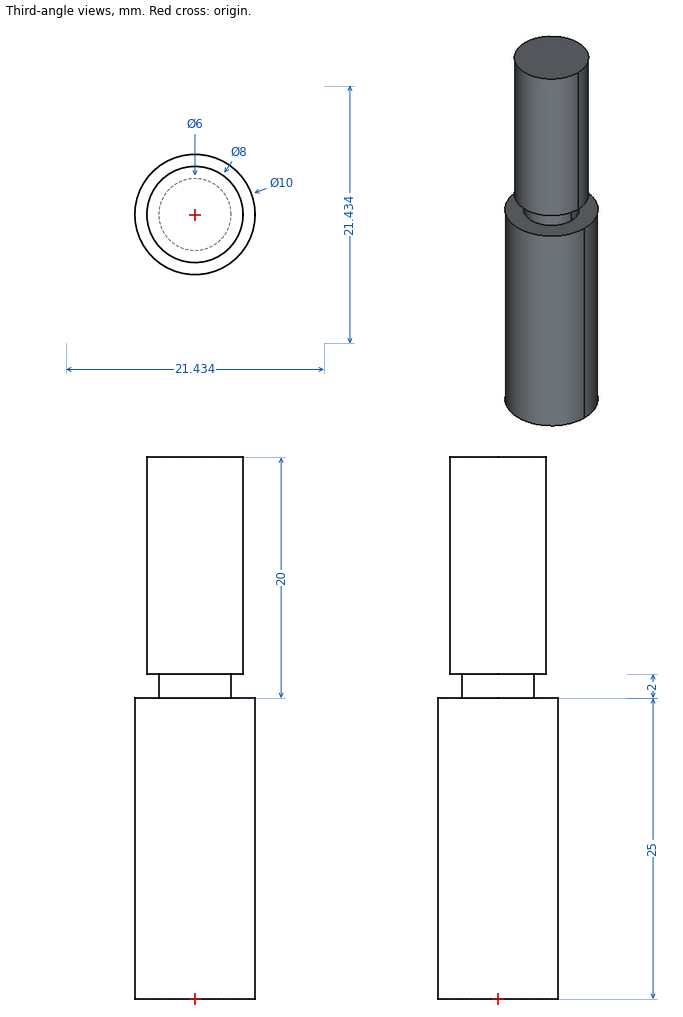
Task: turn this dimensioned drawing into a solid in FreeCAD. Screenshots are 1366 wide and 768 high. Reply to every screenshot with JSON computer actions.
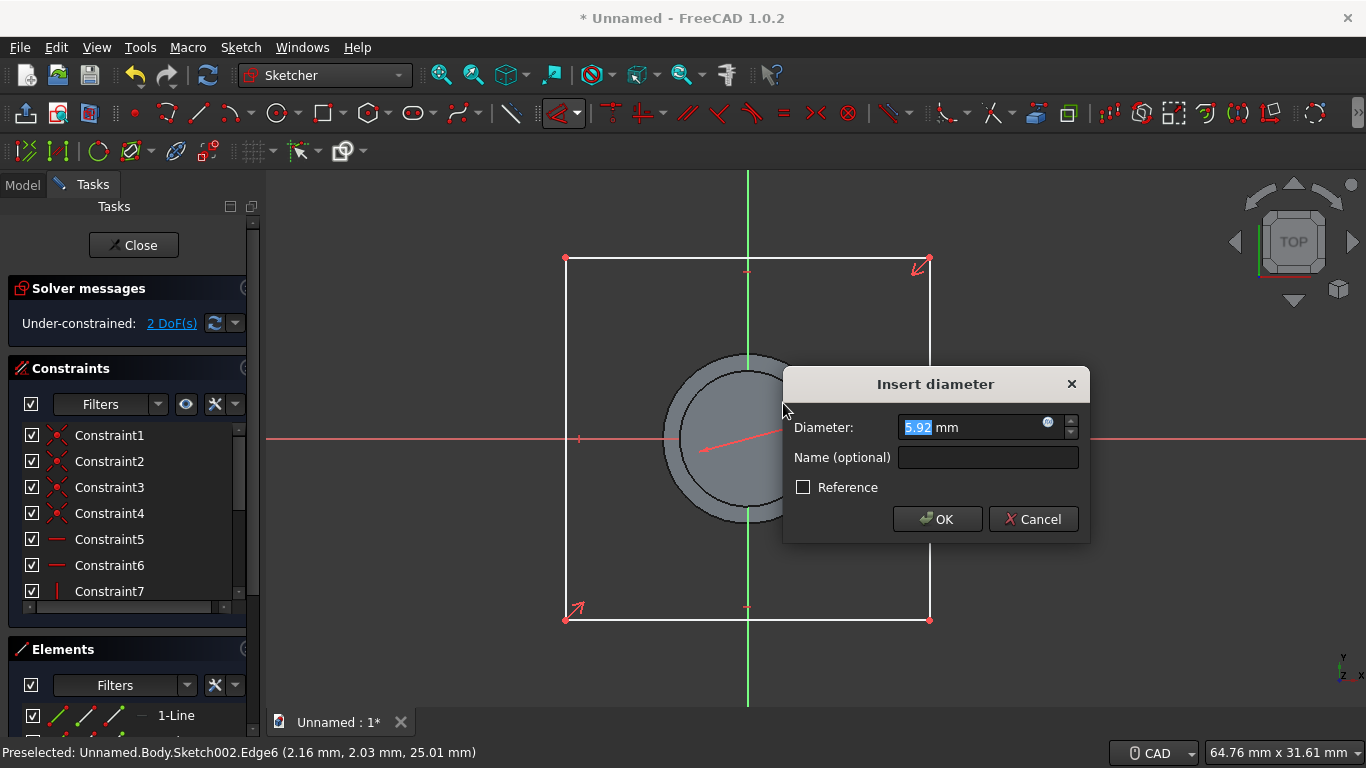
{"action": "type", "text": "6"}
{"action": "key", "text": "Return"}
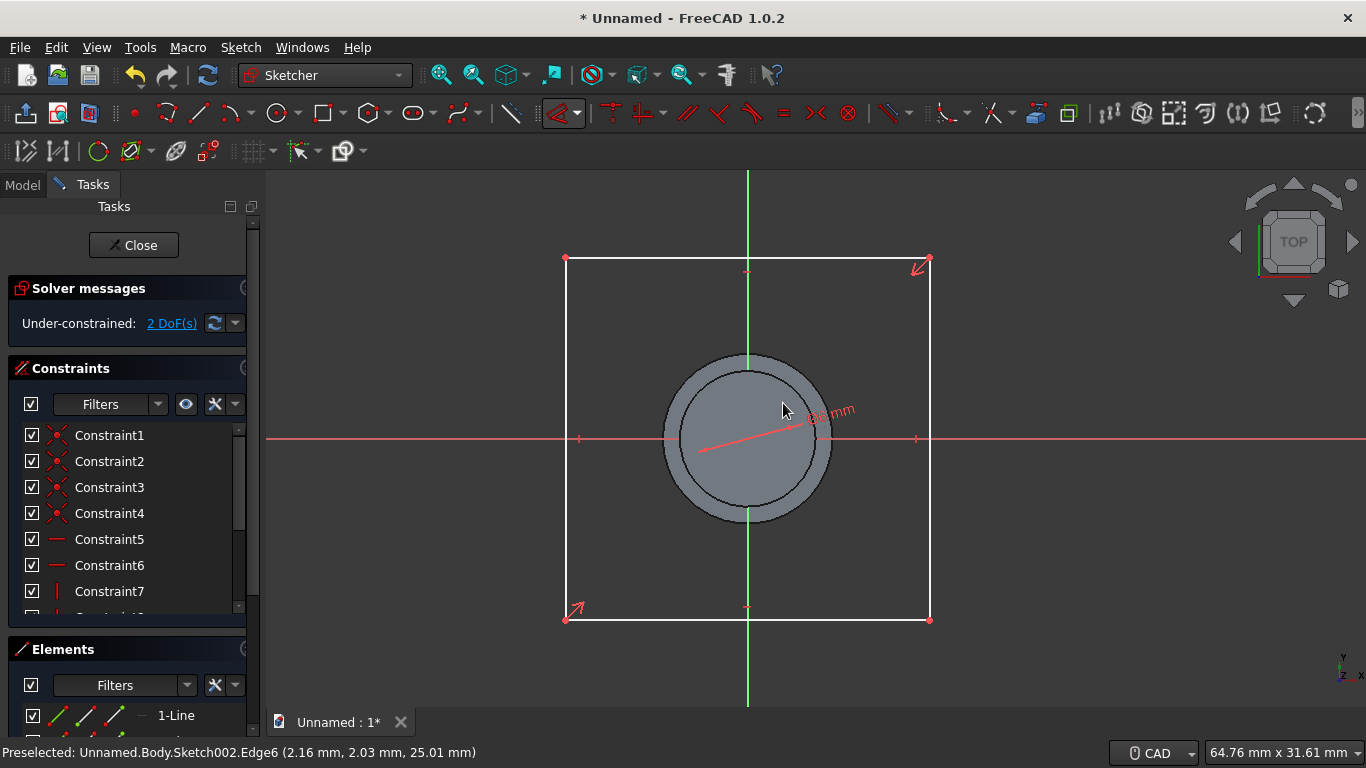
{"action": "left_click", "coordinate": [675, 620]}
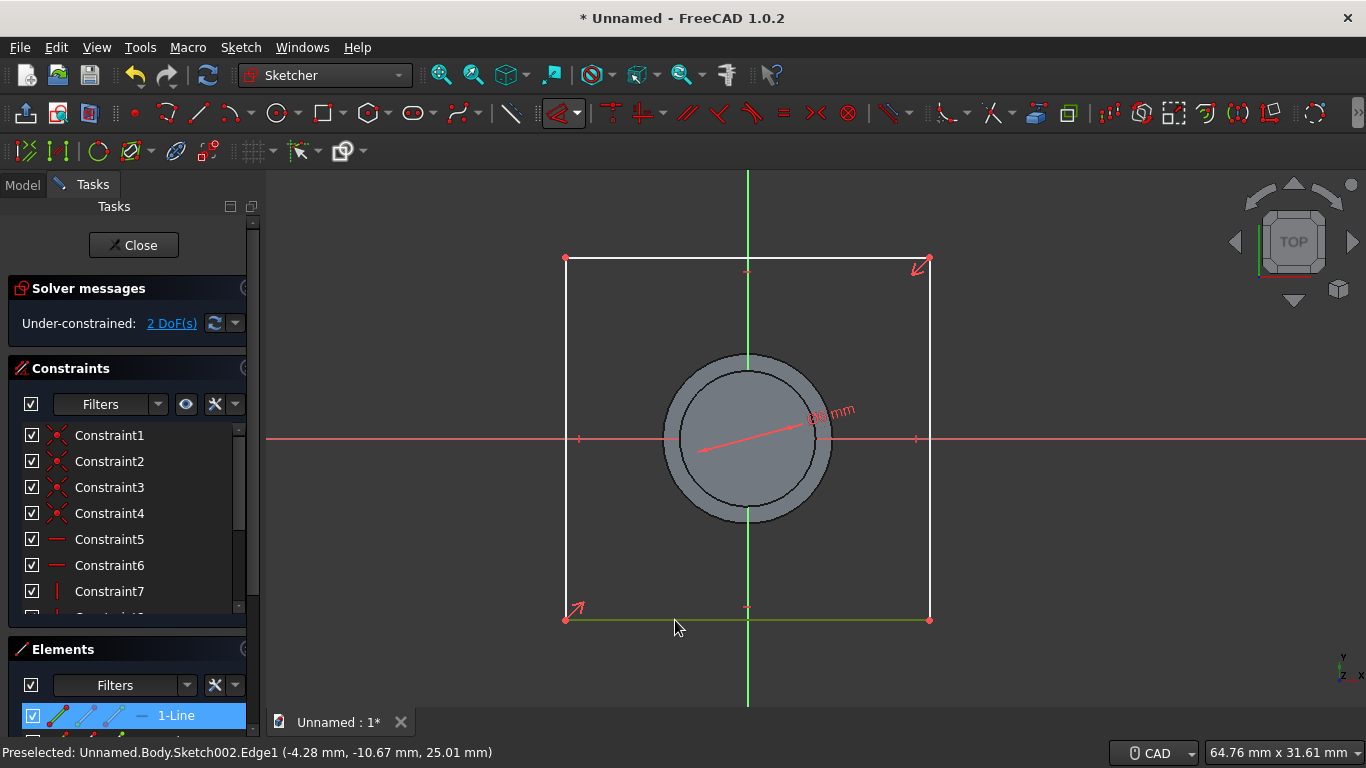
{"action": "left_click", "coordinate": [580, 114]}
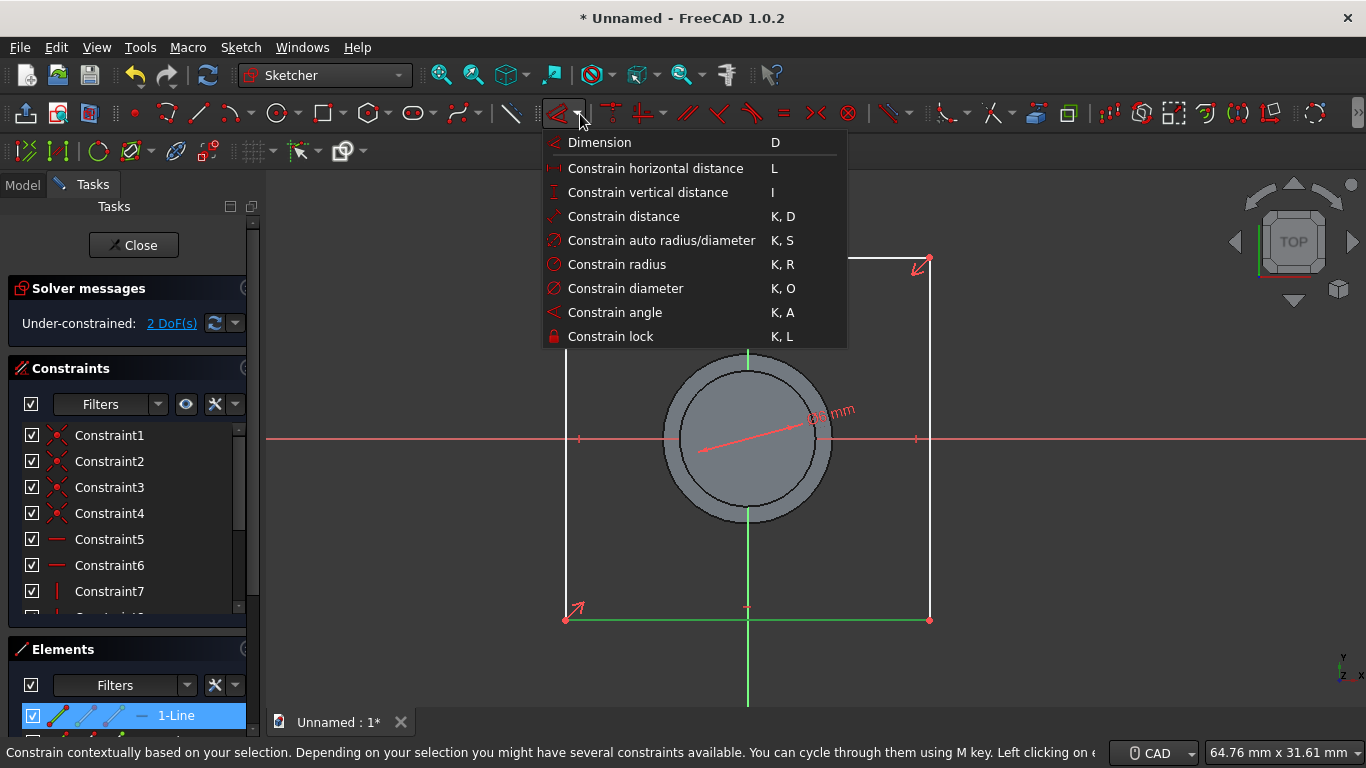
{"action": "left_click", "coordinate": [695, 168]}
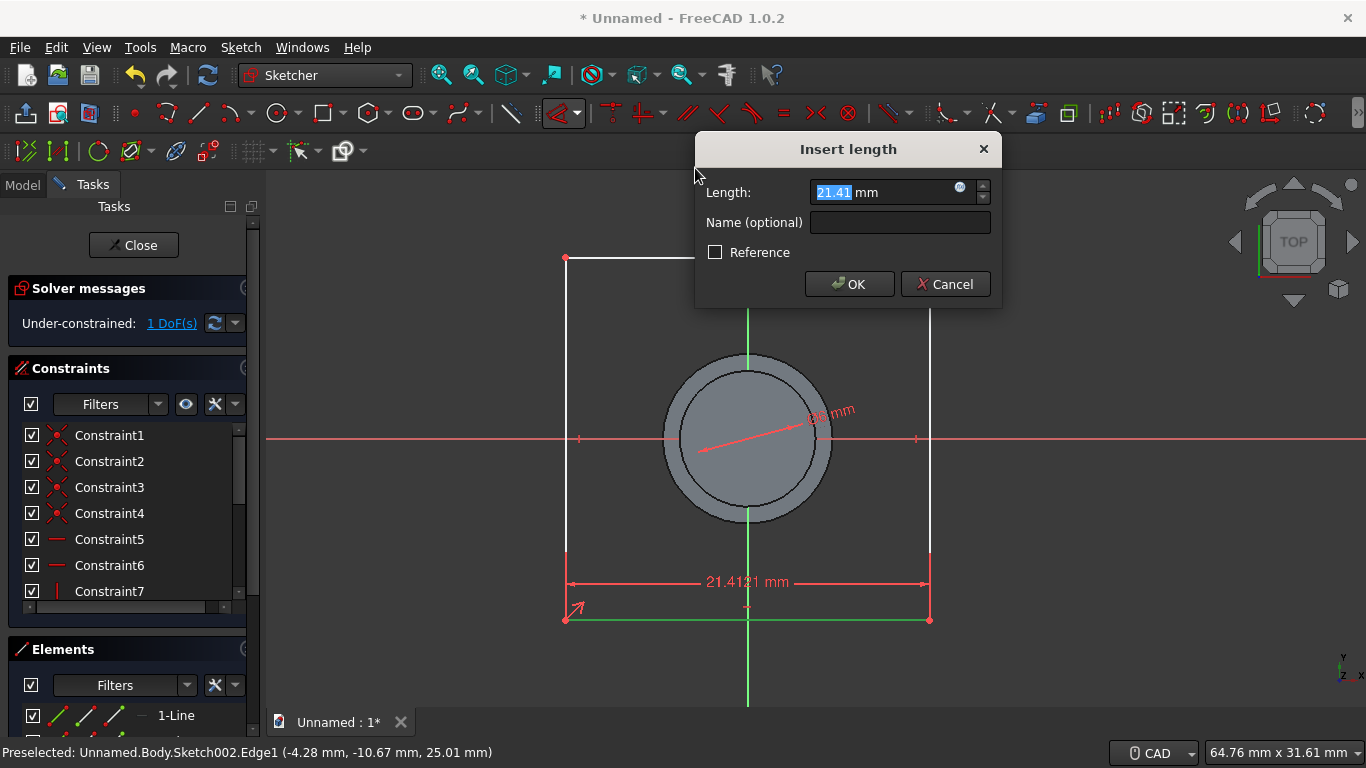
{"action": "type", "text": "21.434"}
{"action": "key", "text": "Return"}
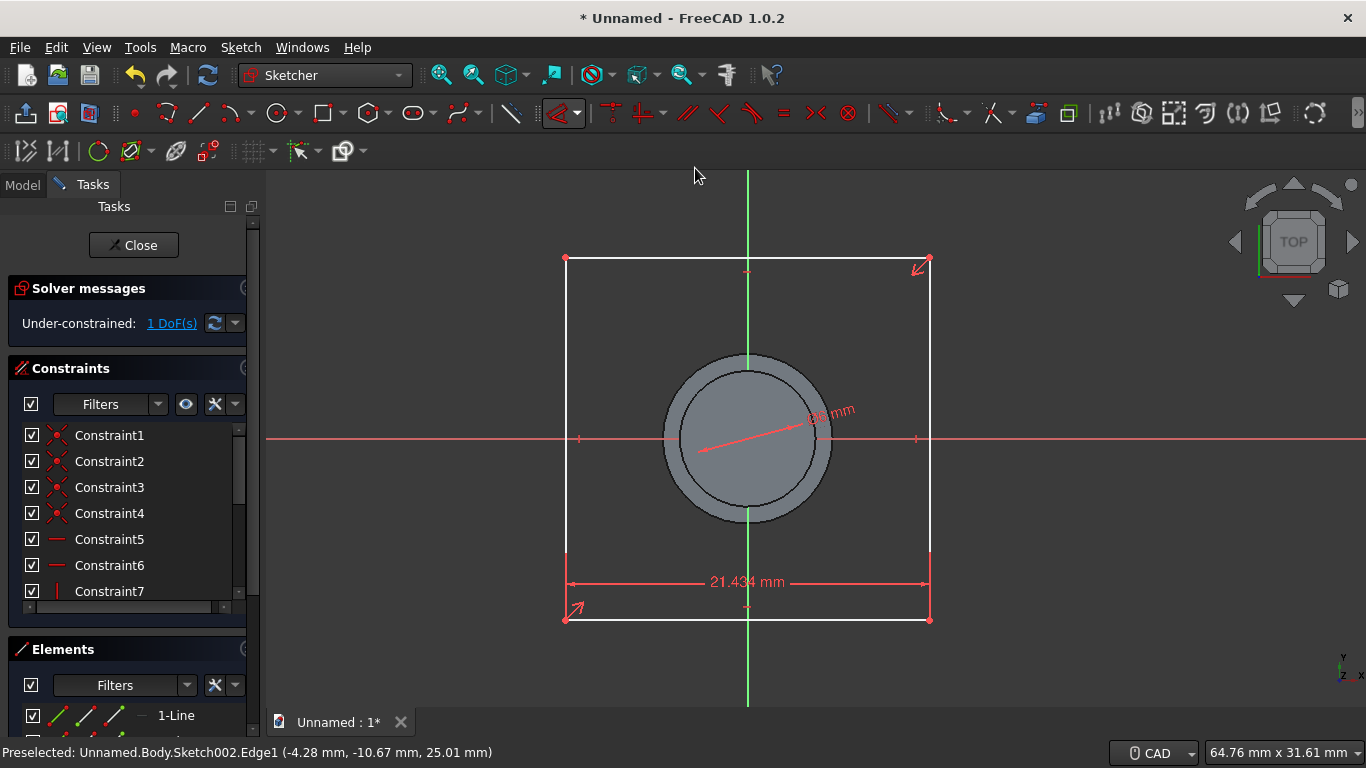
{"action": "left_click", "coordinate": [930, 511]}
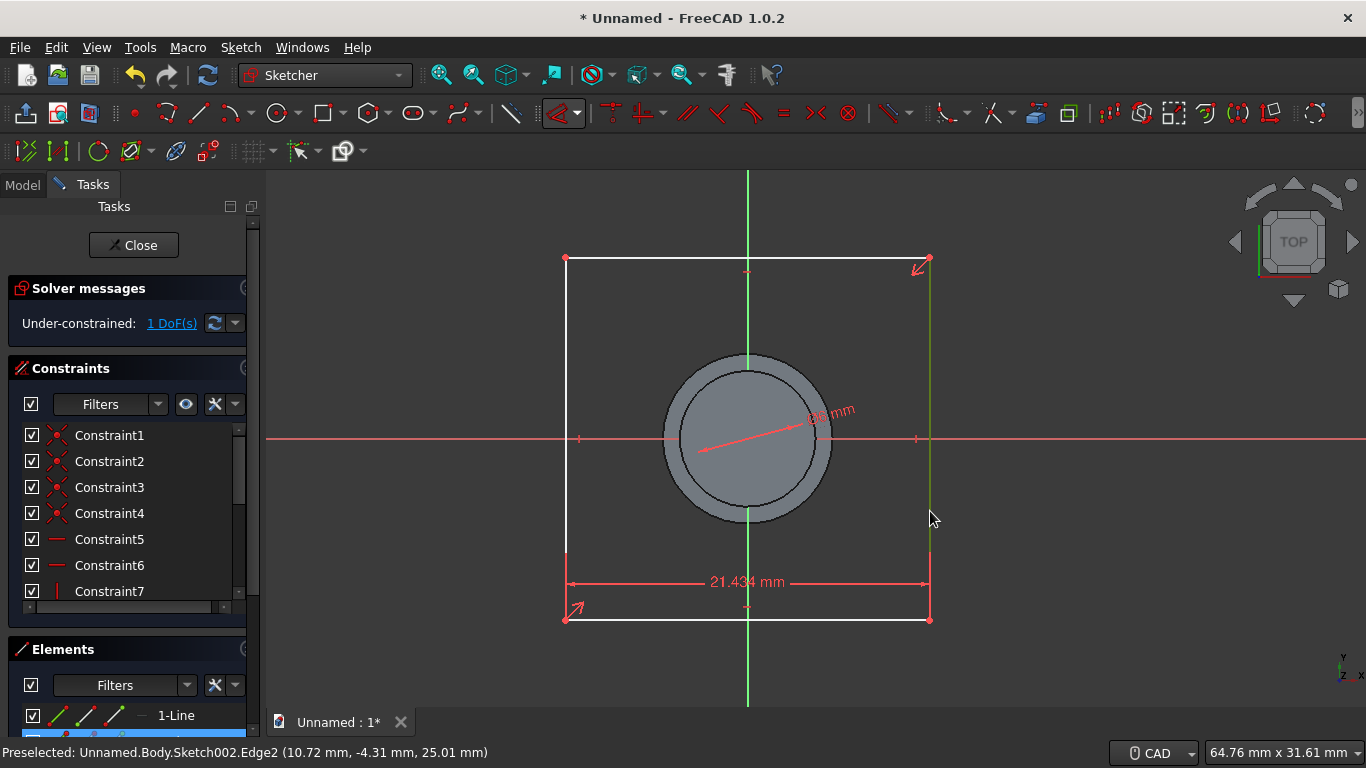
{"action": "left_click", "coordinate": [580, 114]}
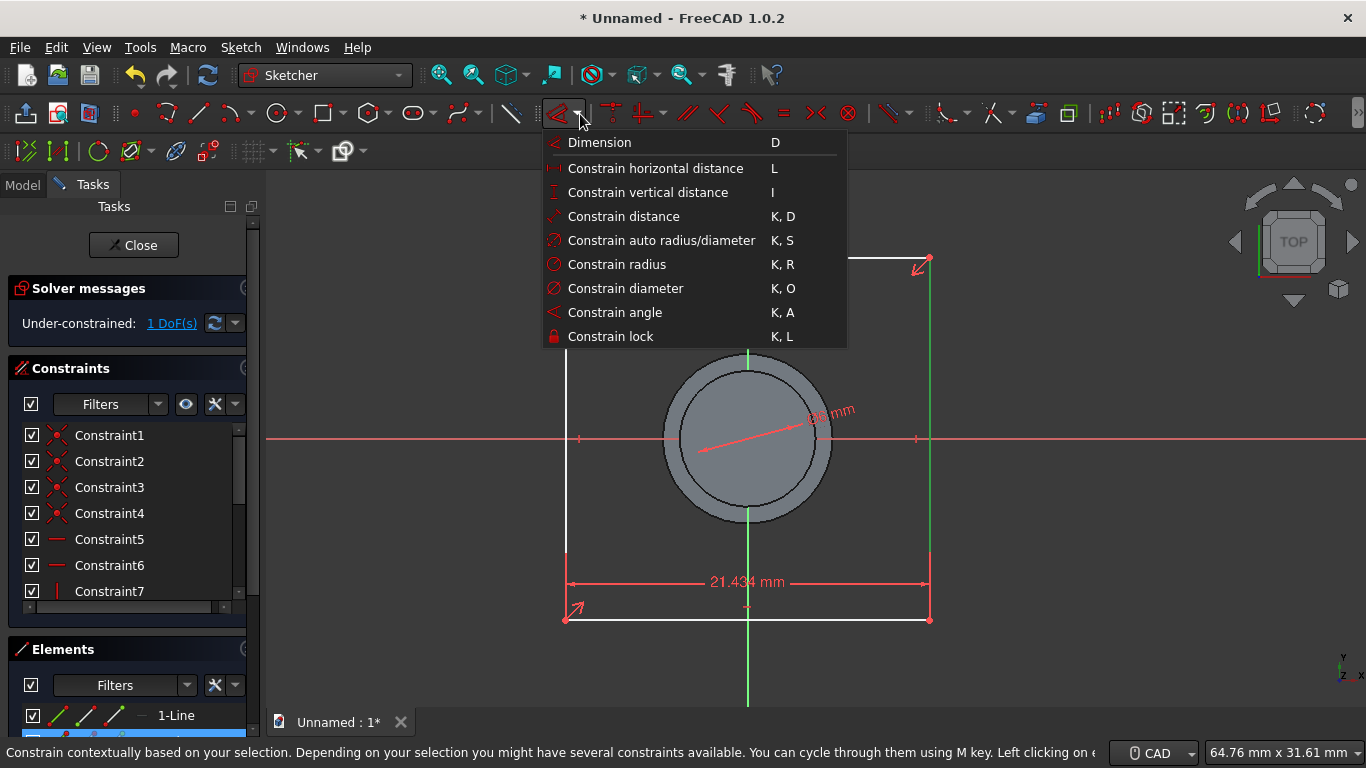
{"action": "left_click", "coordinate": [695, 192]}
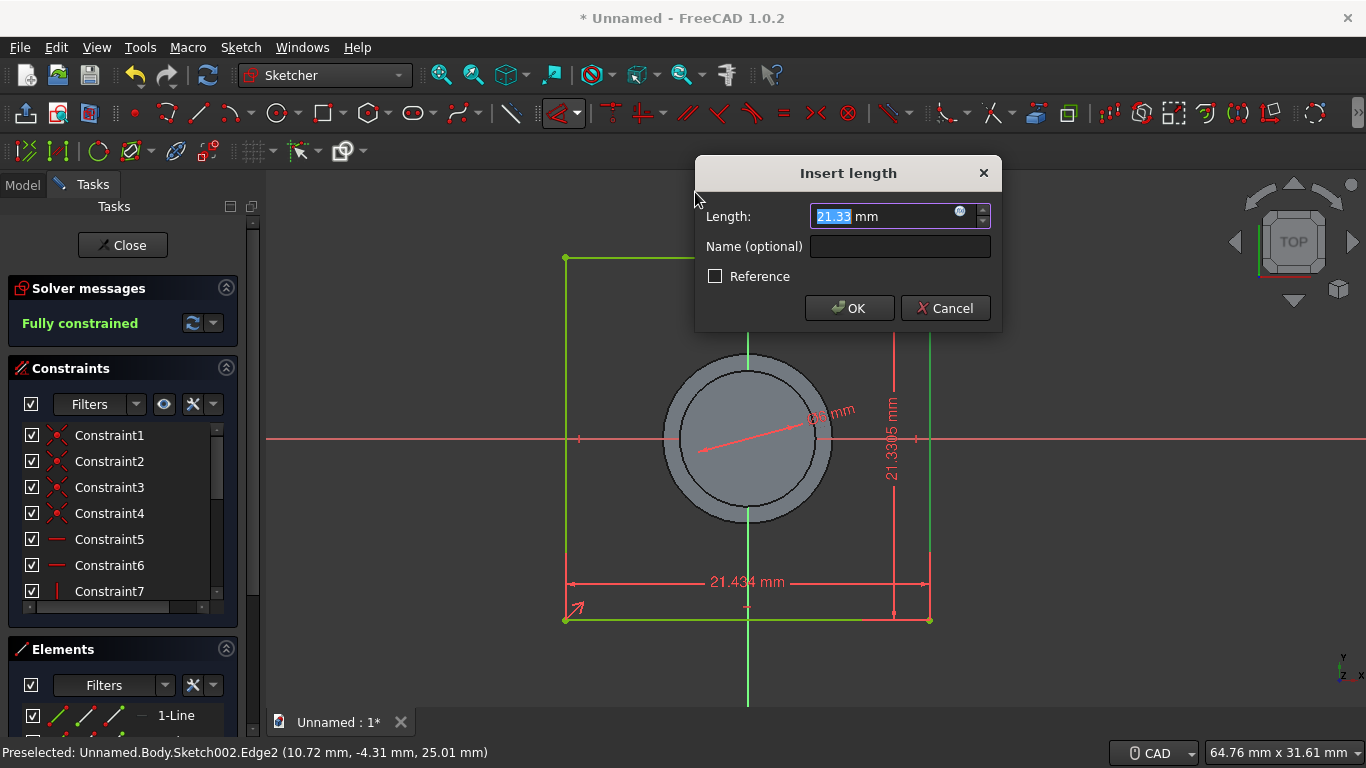
{"action": "type", "text": "21.434"}
{"action": "key", "text": "Return"}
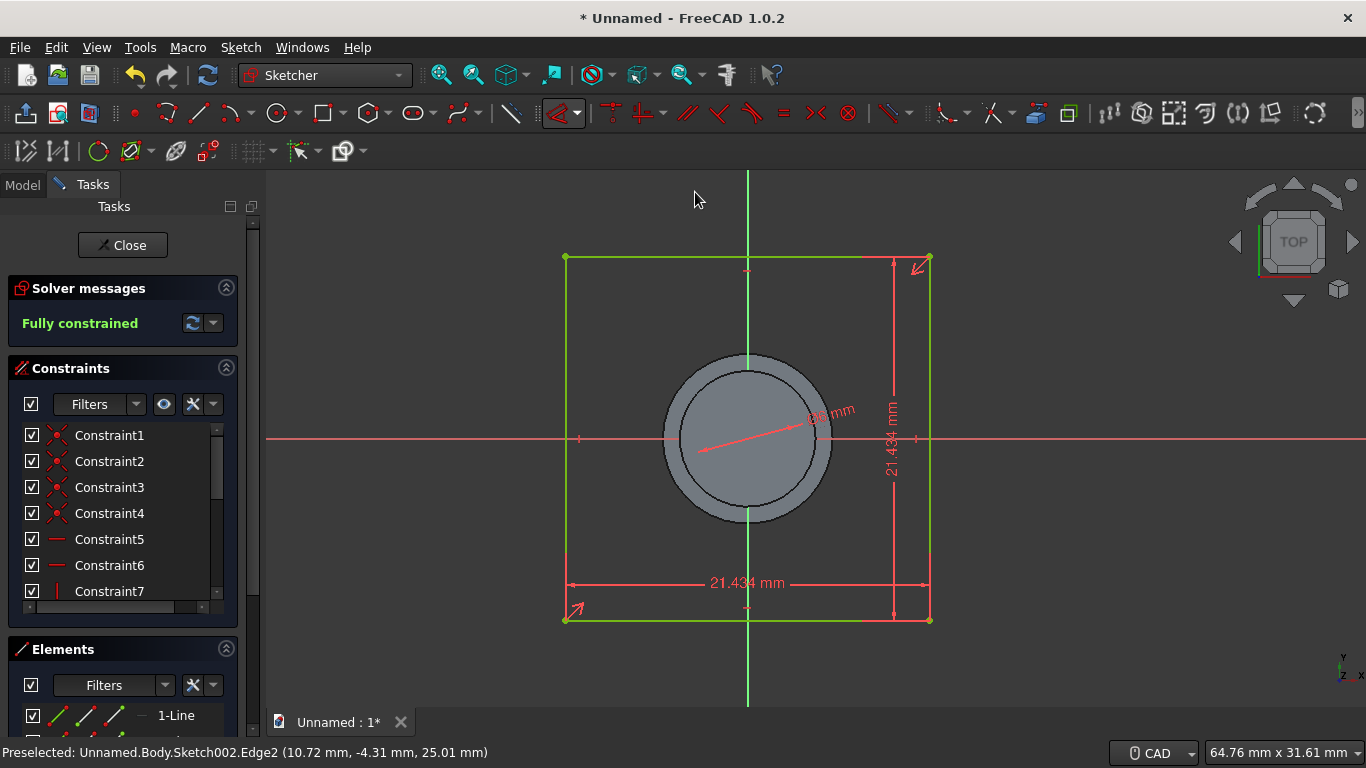
{"action": "left_click", "coordinate": [123, 245]}